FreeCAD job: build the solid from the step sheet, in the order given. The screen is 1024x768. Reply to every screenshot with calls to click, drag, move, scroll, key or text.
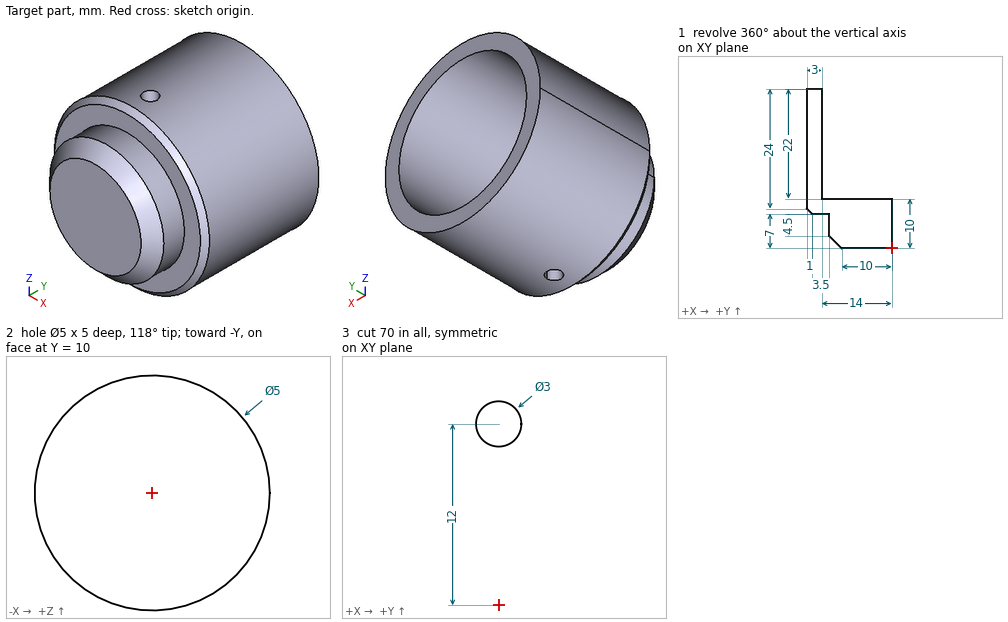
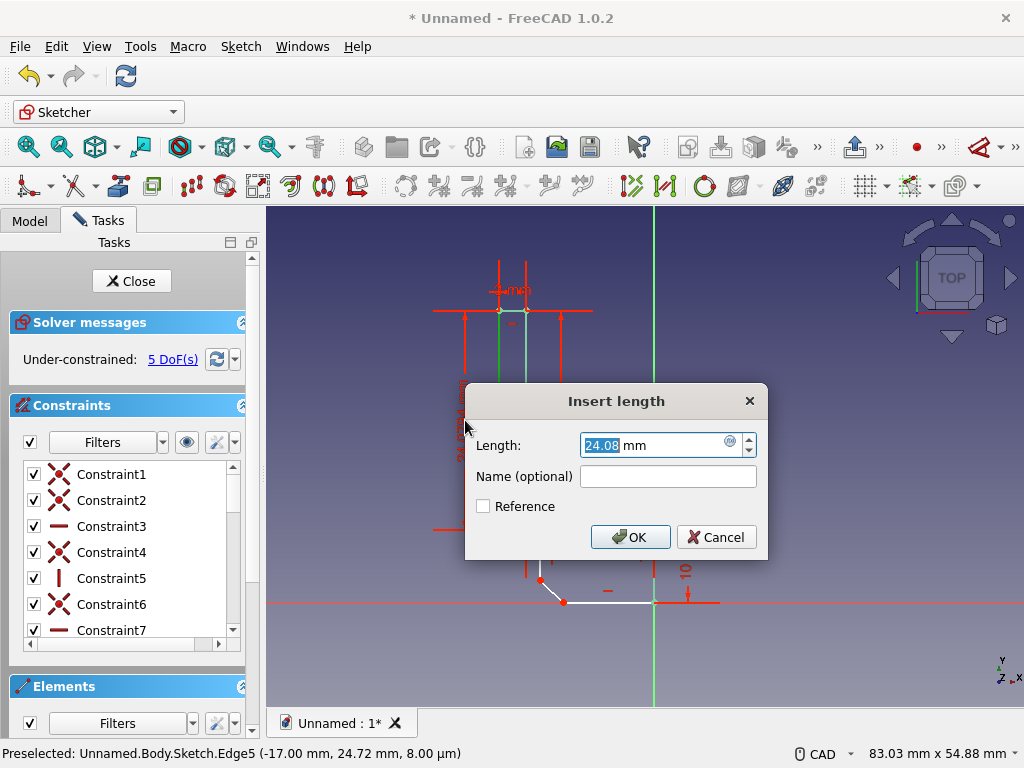
text(24)
key(Return)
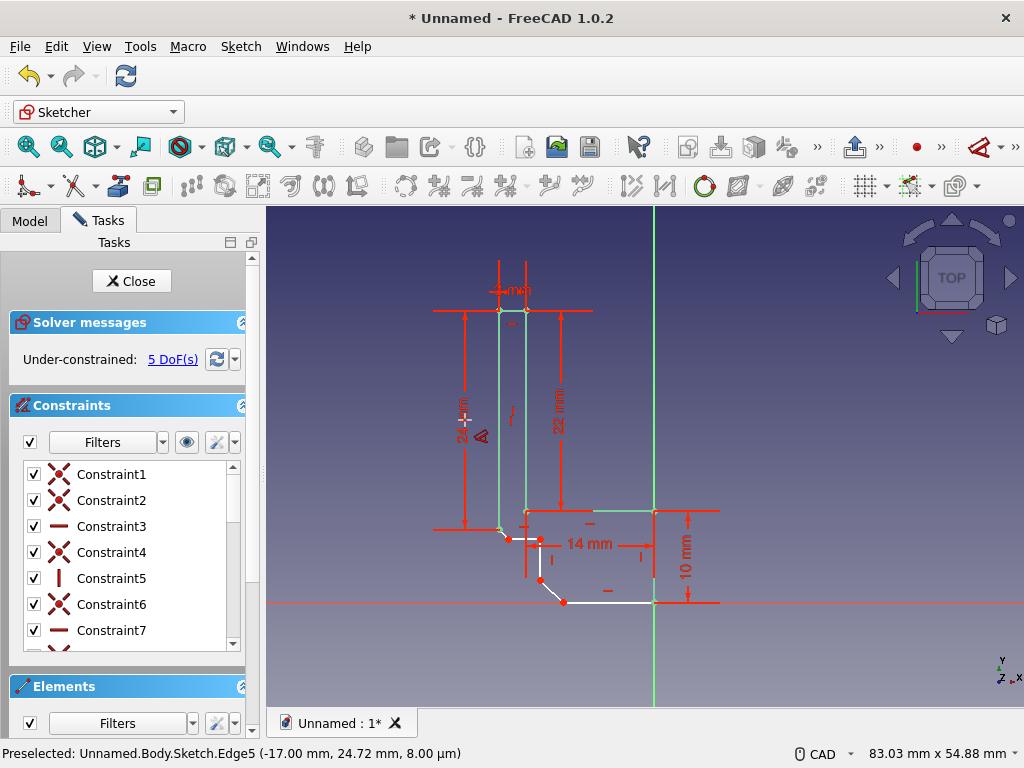
click(590, 603)
click(609, 637)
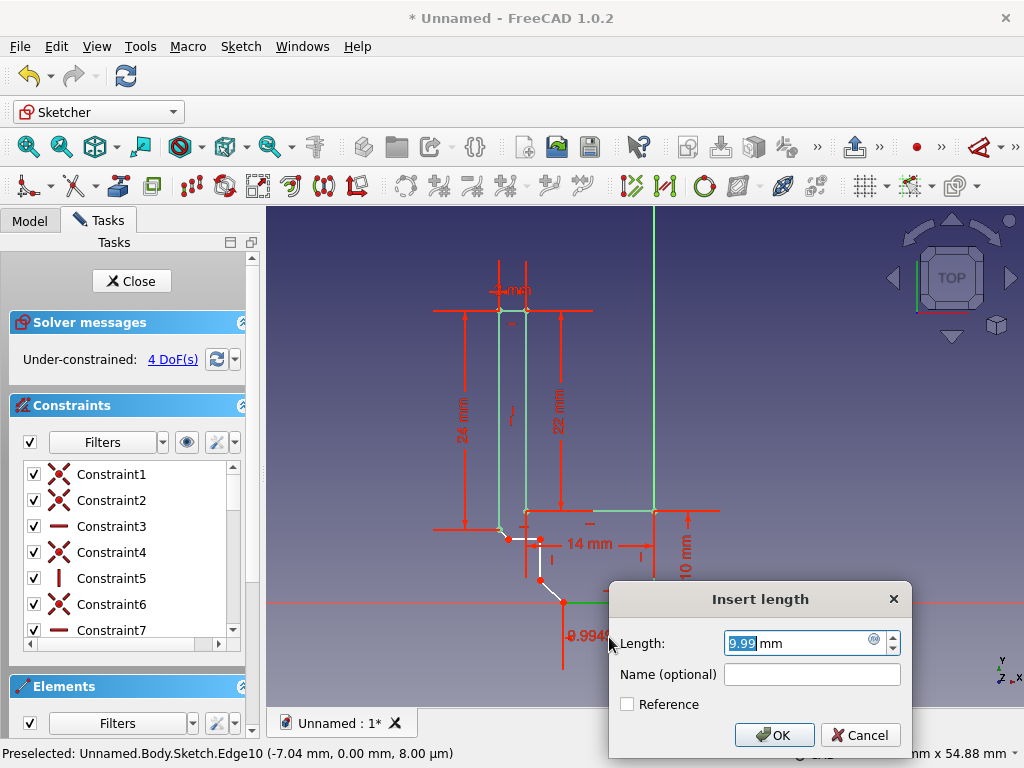
text(10)
key(Return)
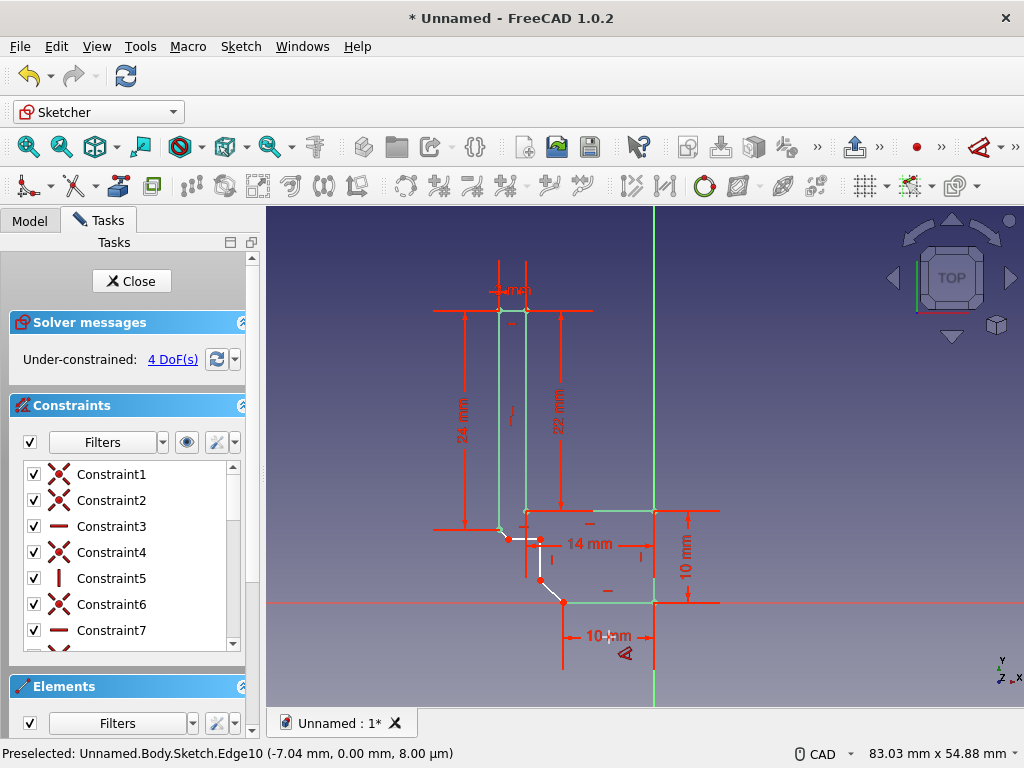
click(508, 539)
click(688, 586)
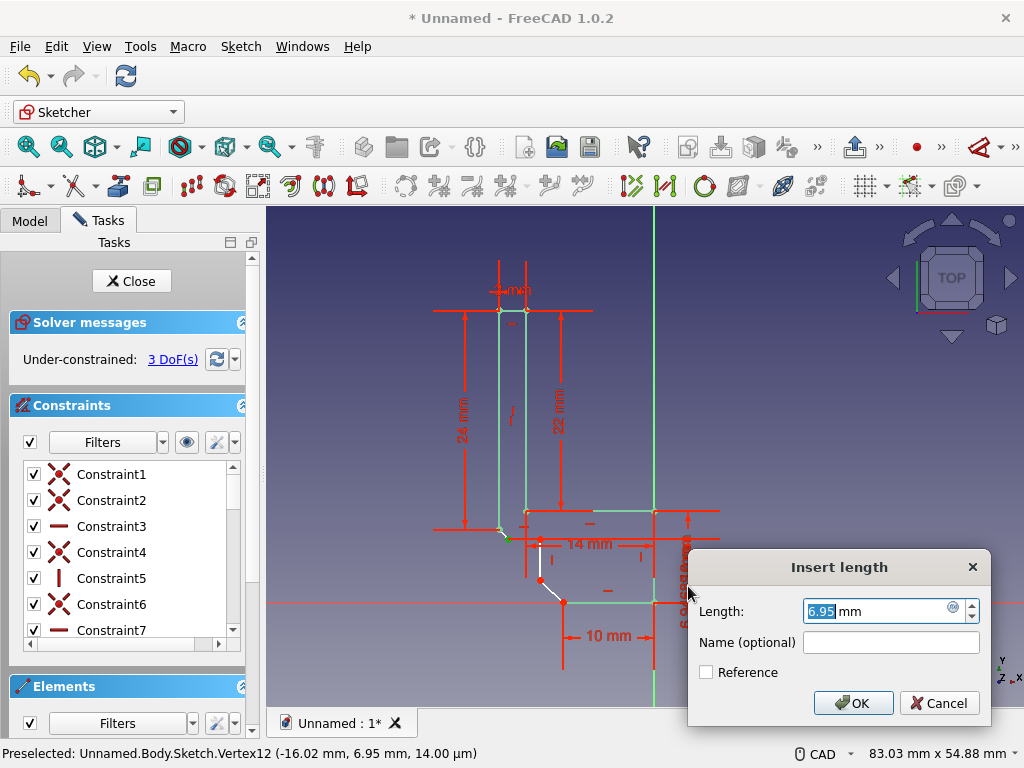
text(7)
key(Return)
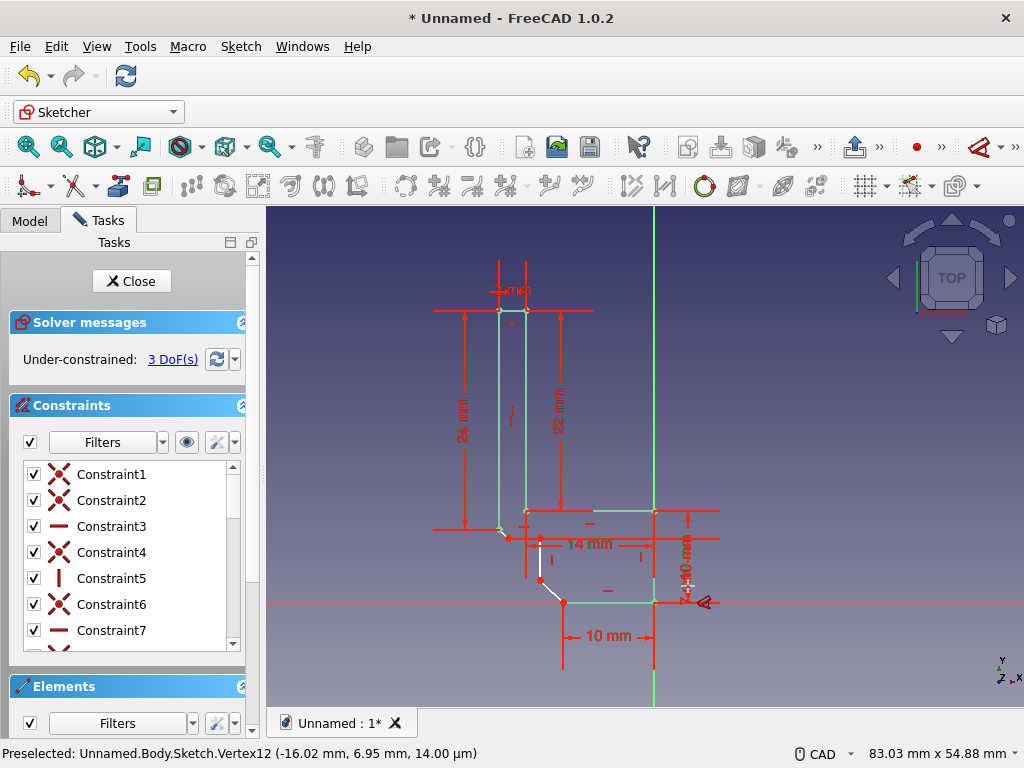
scroll(504, 534, up, 8)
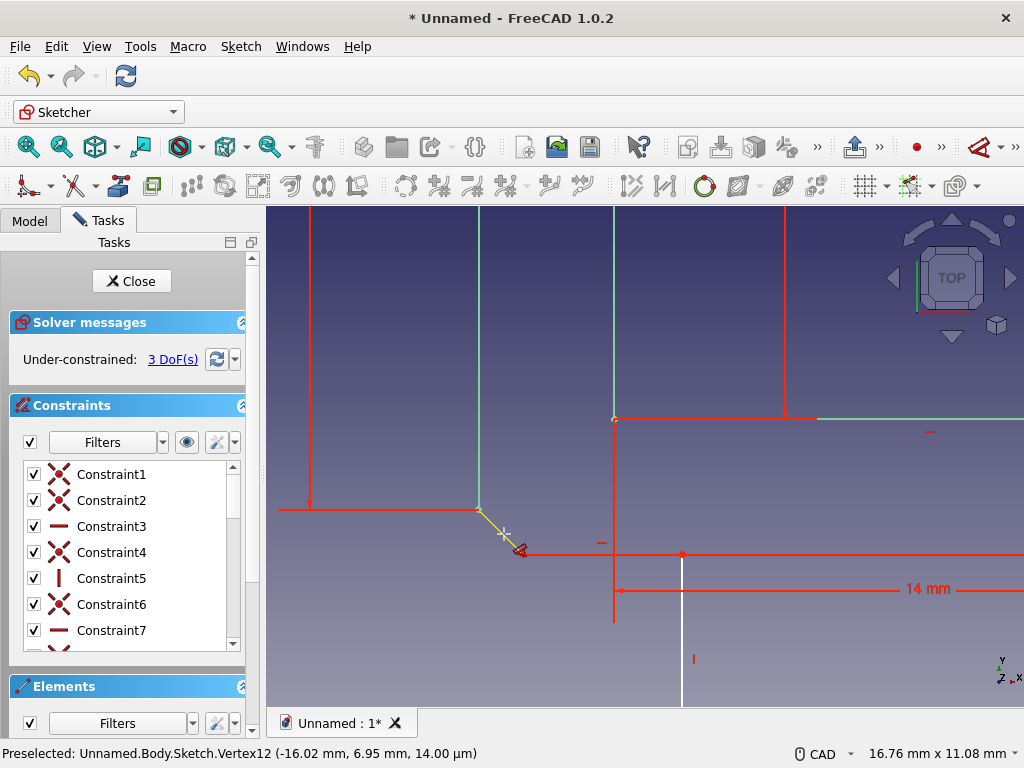
click(501, 532)
click(501, 589)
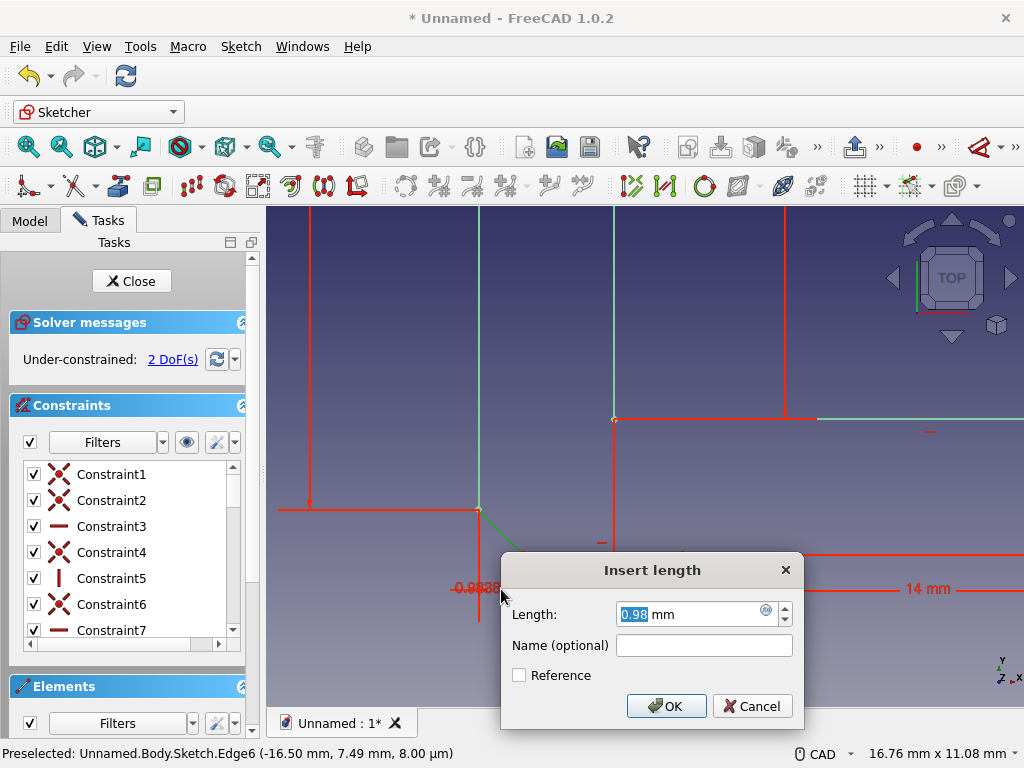
text(1)
key(Return)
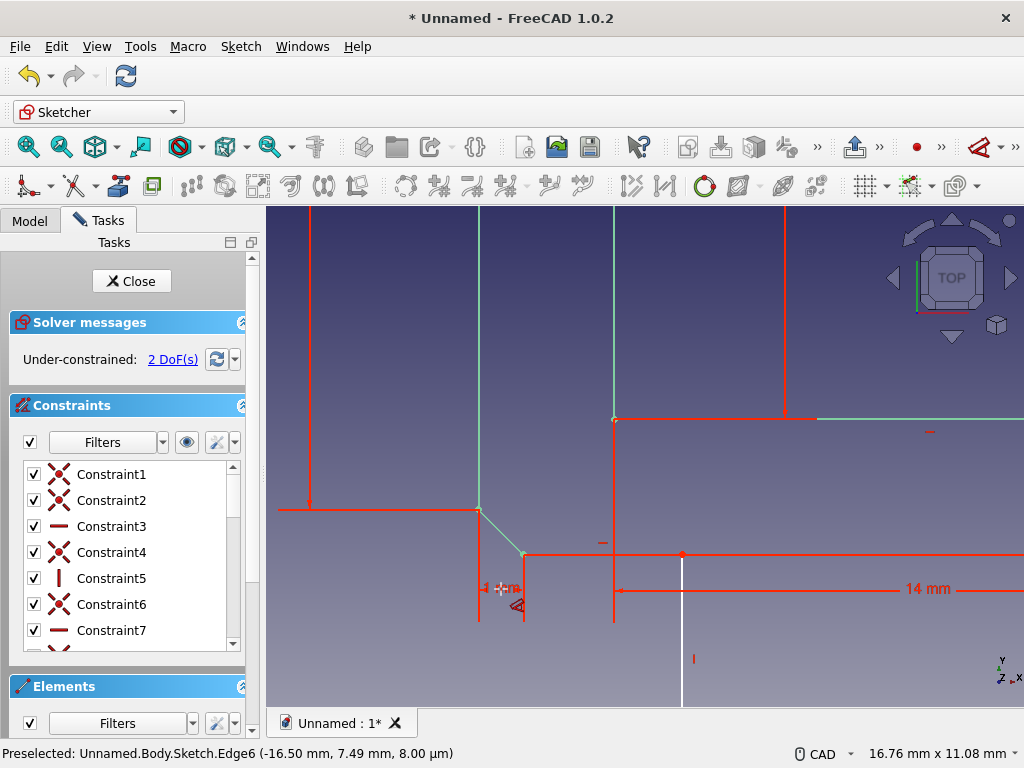
scroll(504, 535, down, 8)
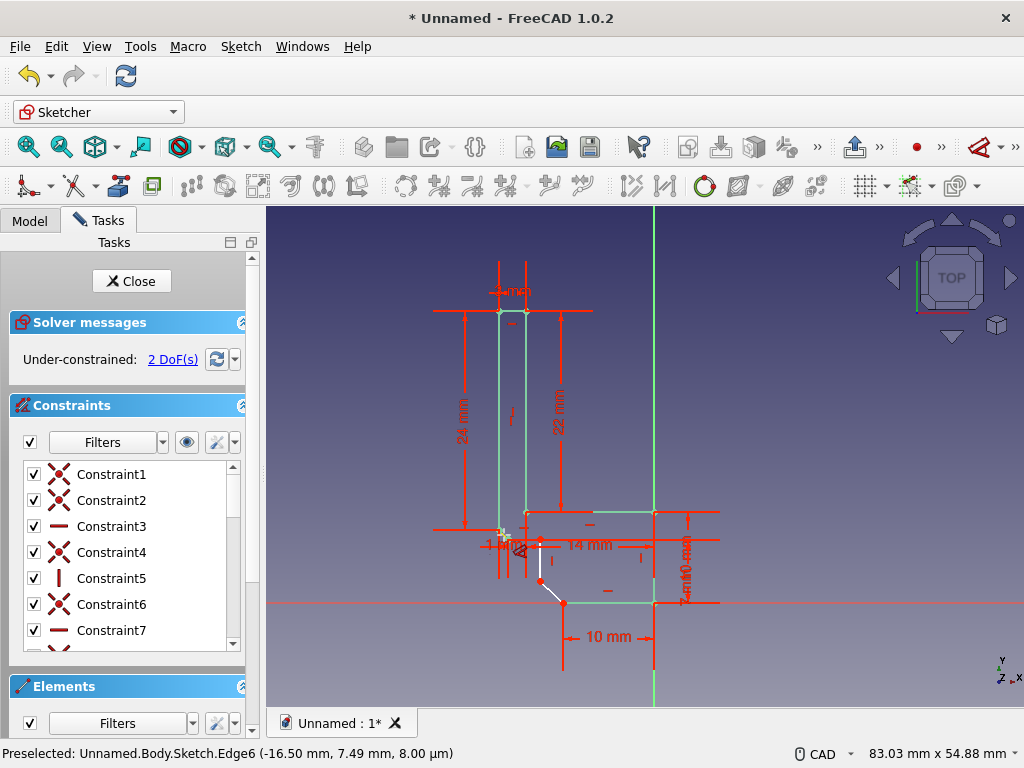
scroll(518, 540, up, 2)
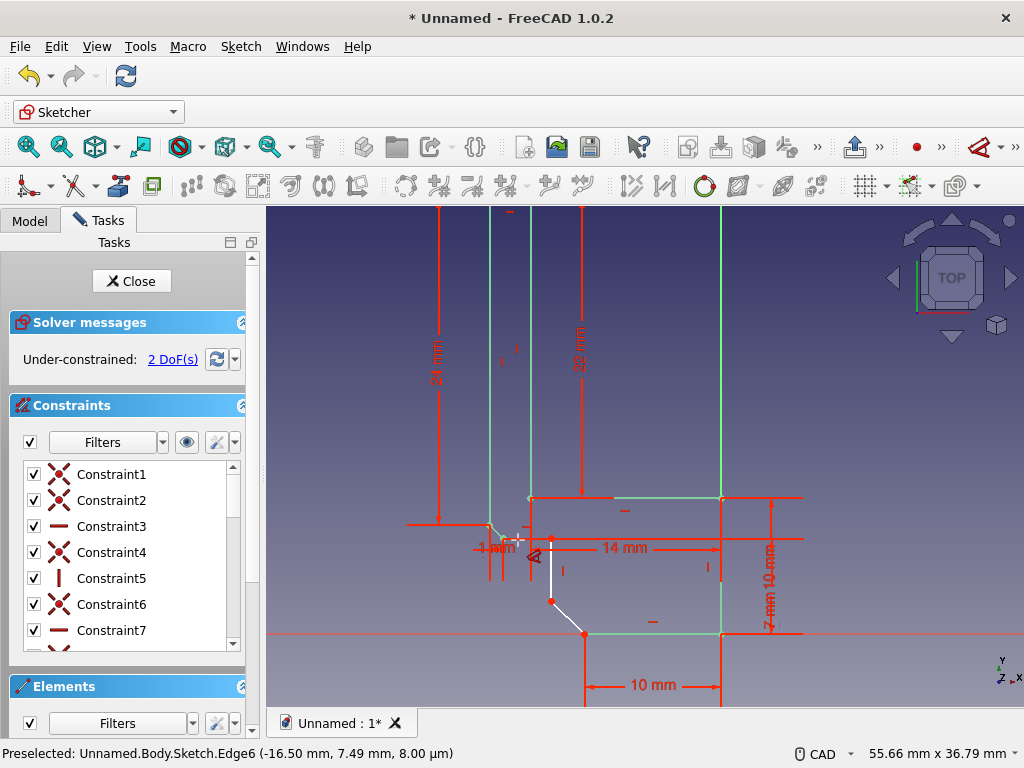
click(518, 539)
click(527, 573)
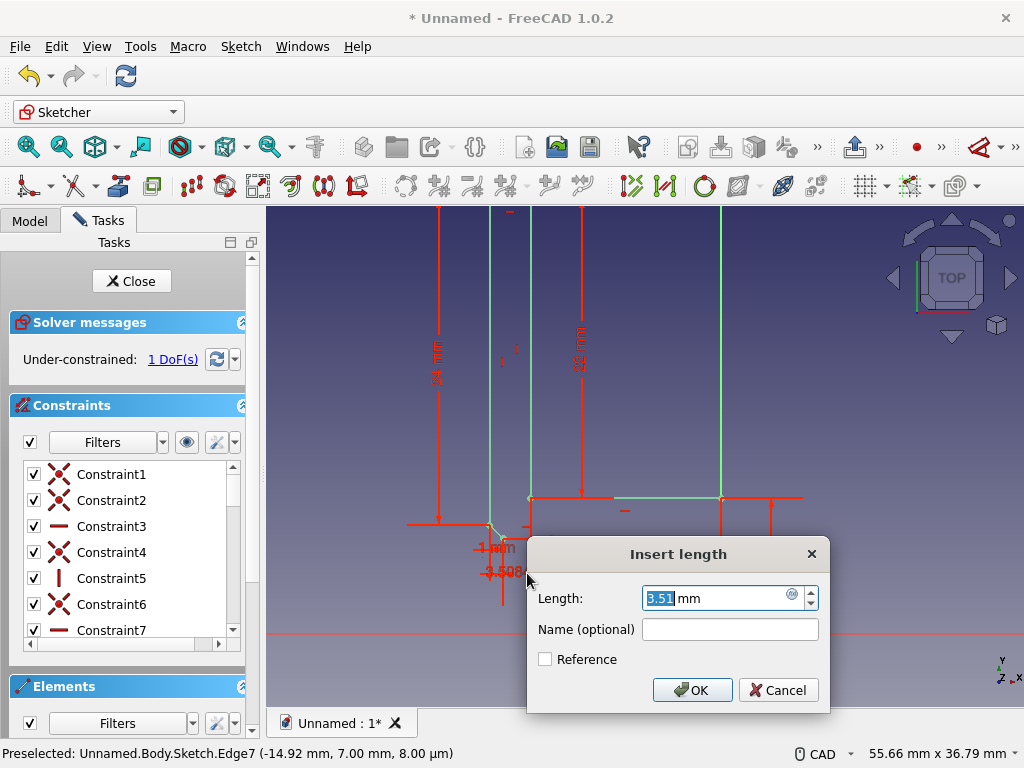
text(3.5)
key(Return)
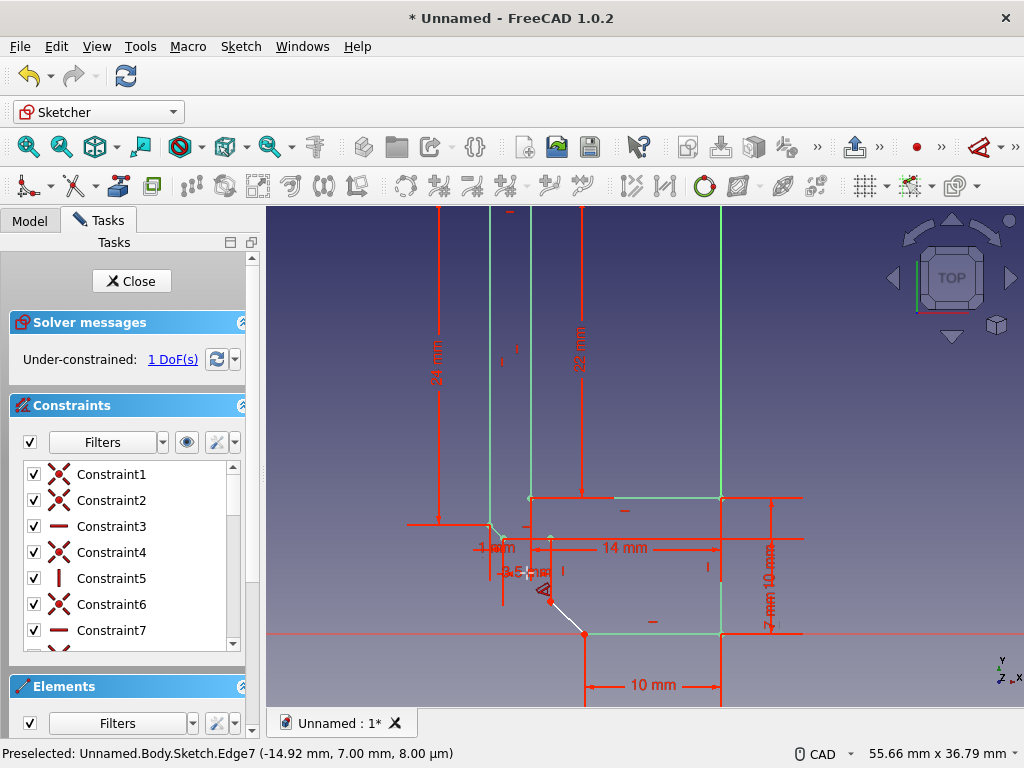
click(551, 558)
click(609, 570)